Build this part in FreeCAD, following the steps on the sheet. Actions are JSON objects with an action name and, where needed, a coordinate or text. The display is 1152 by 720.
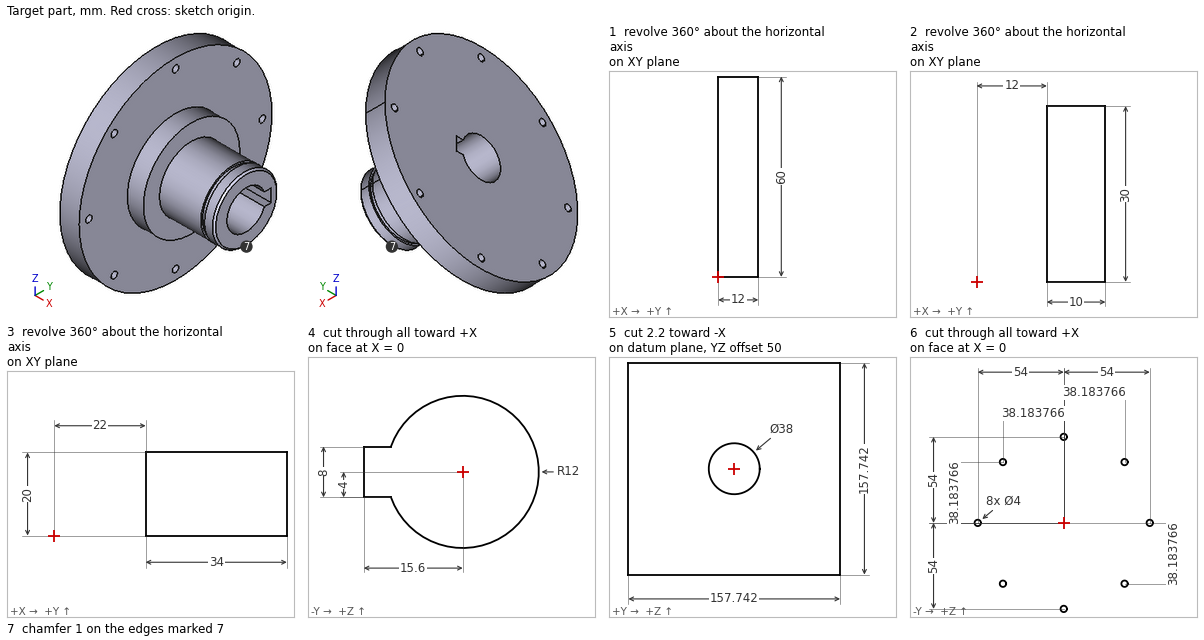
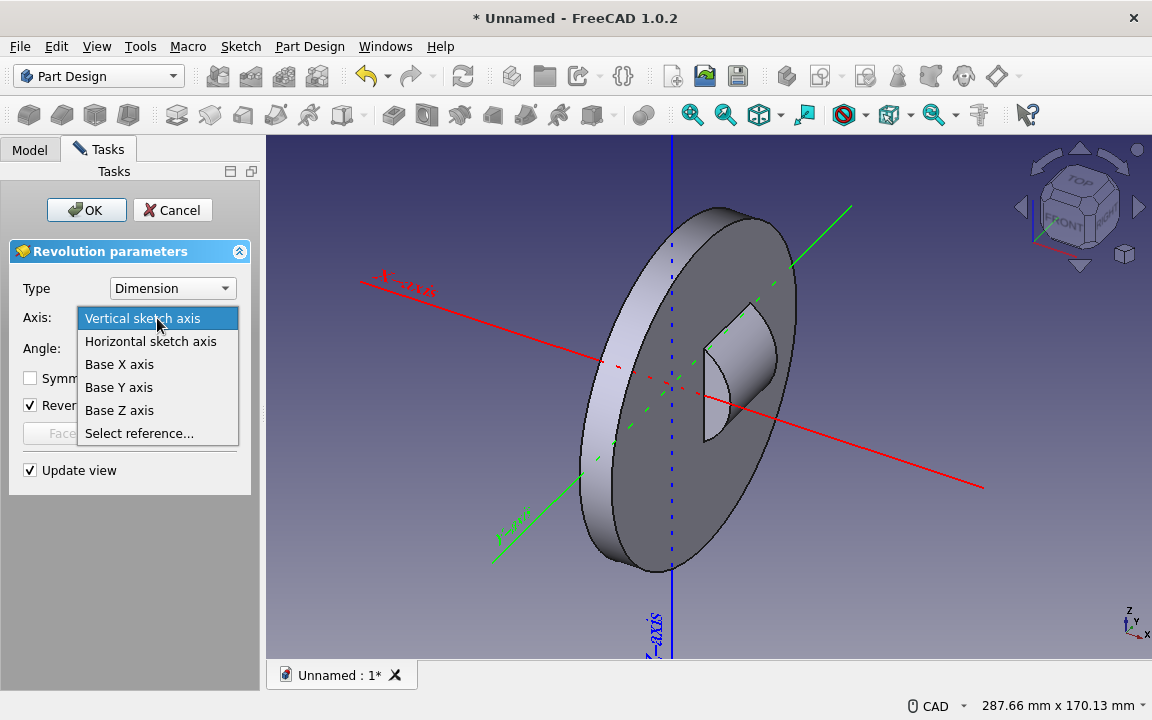
{"action": "left_click", "coordinate": [156, 342]}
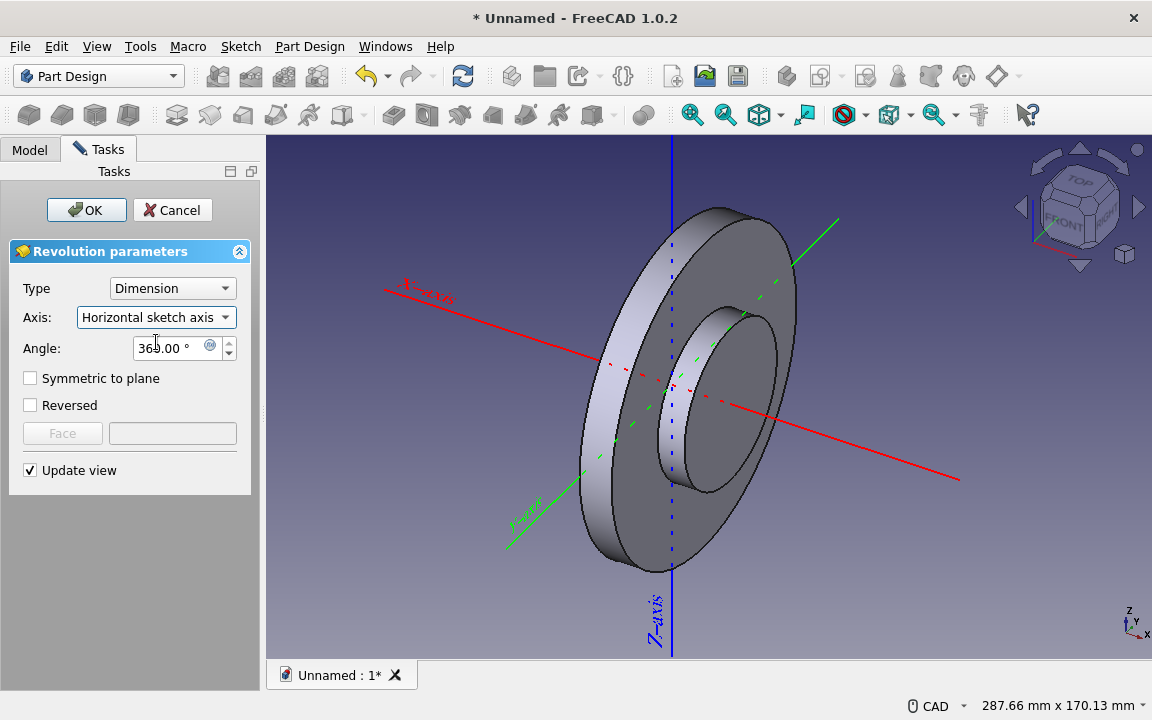
{"action": "left_click", "coordinate": [87, 210]}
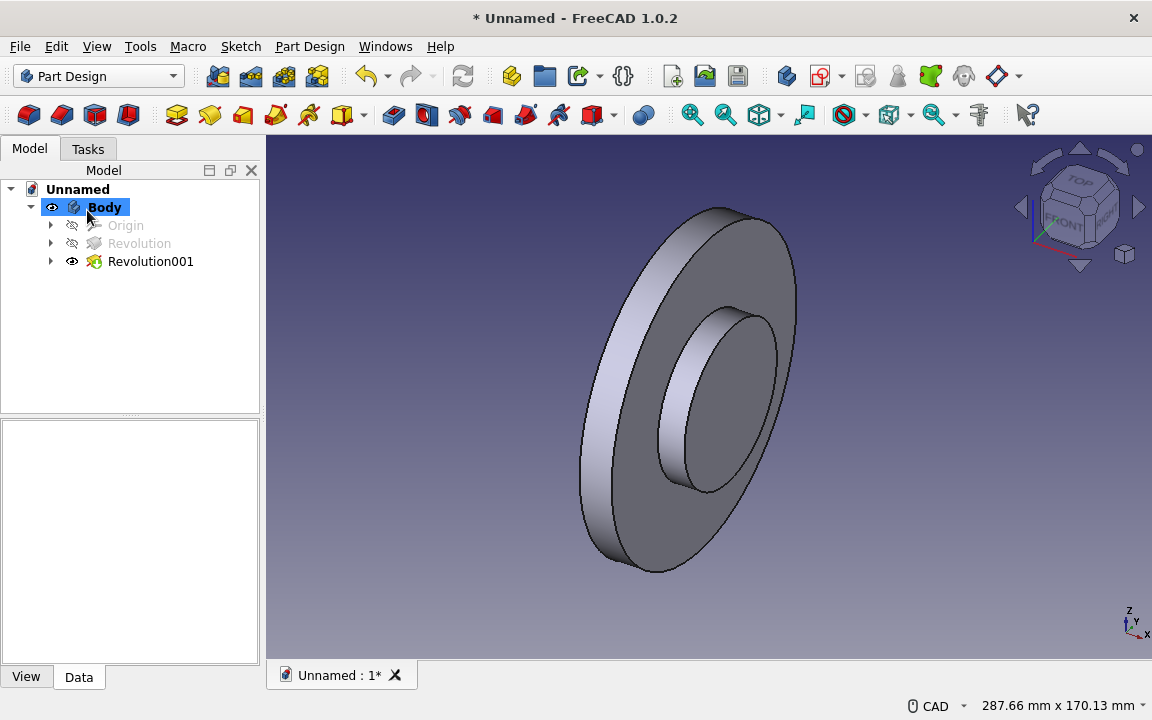
{"action": "left_click", "coordinate": [820, 76]}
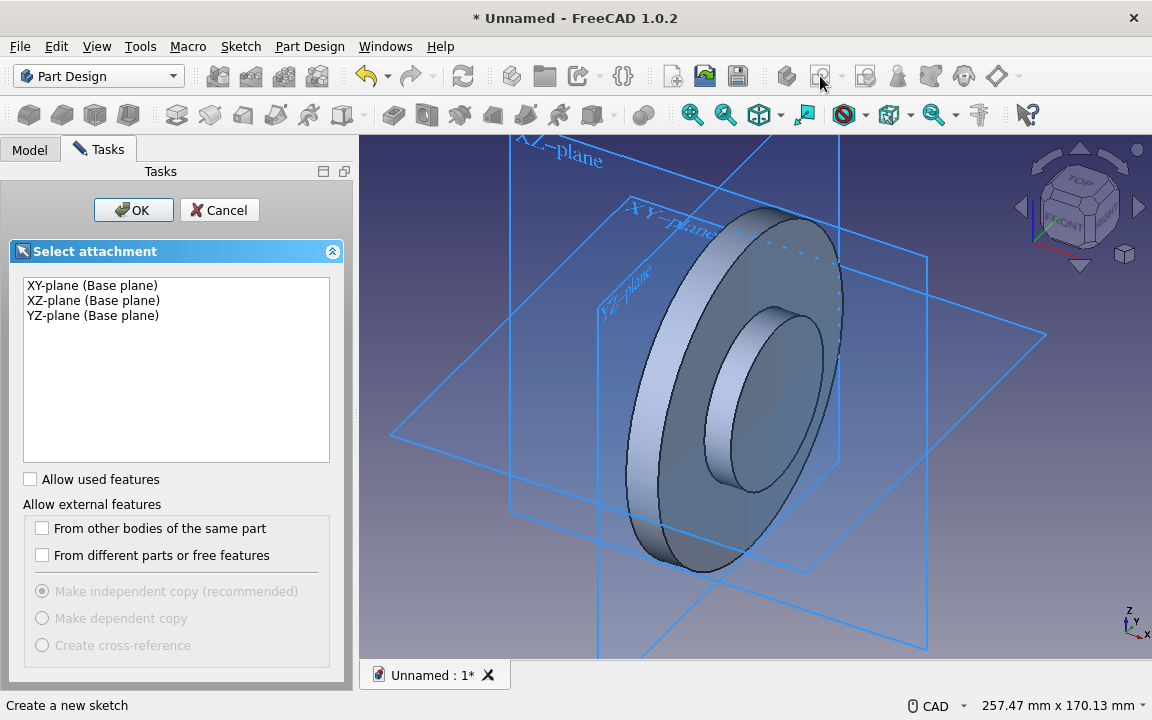
{"action": "left_click", "coordinate": [84, 286]}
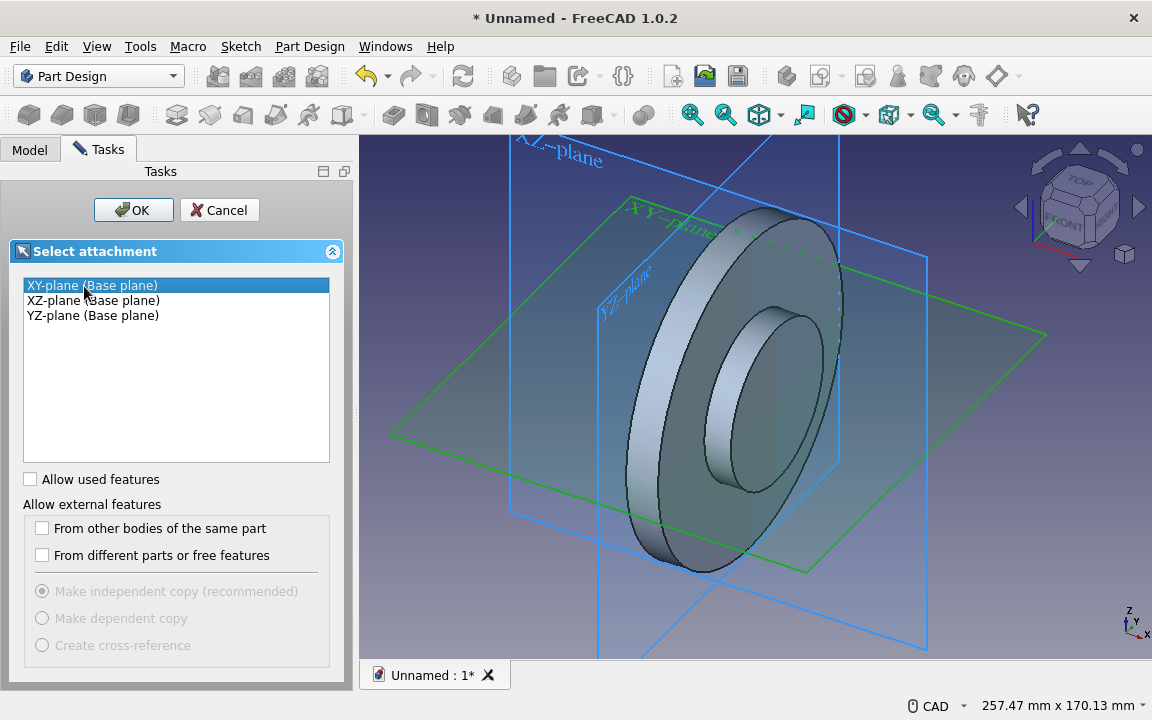
{"action": "left_click", "coordinate": [134, 210]}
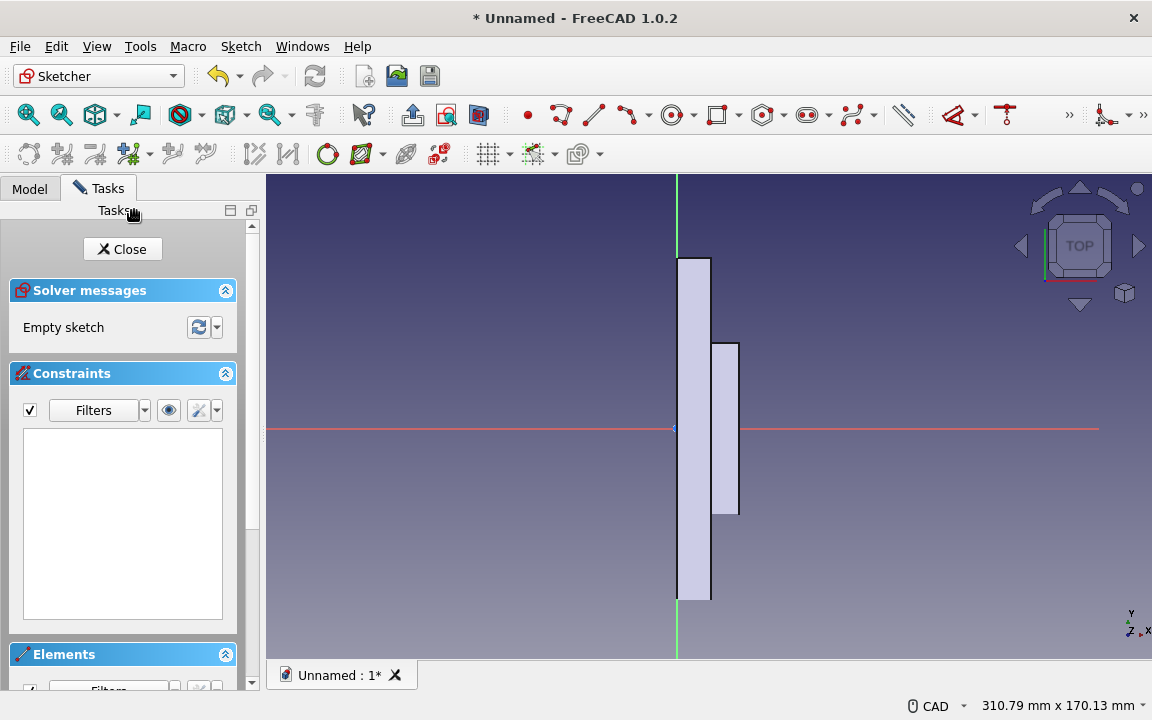
{"action": "left_click", "coordinate": [479, 116]}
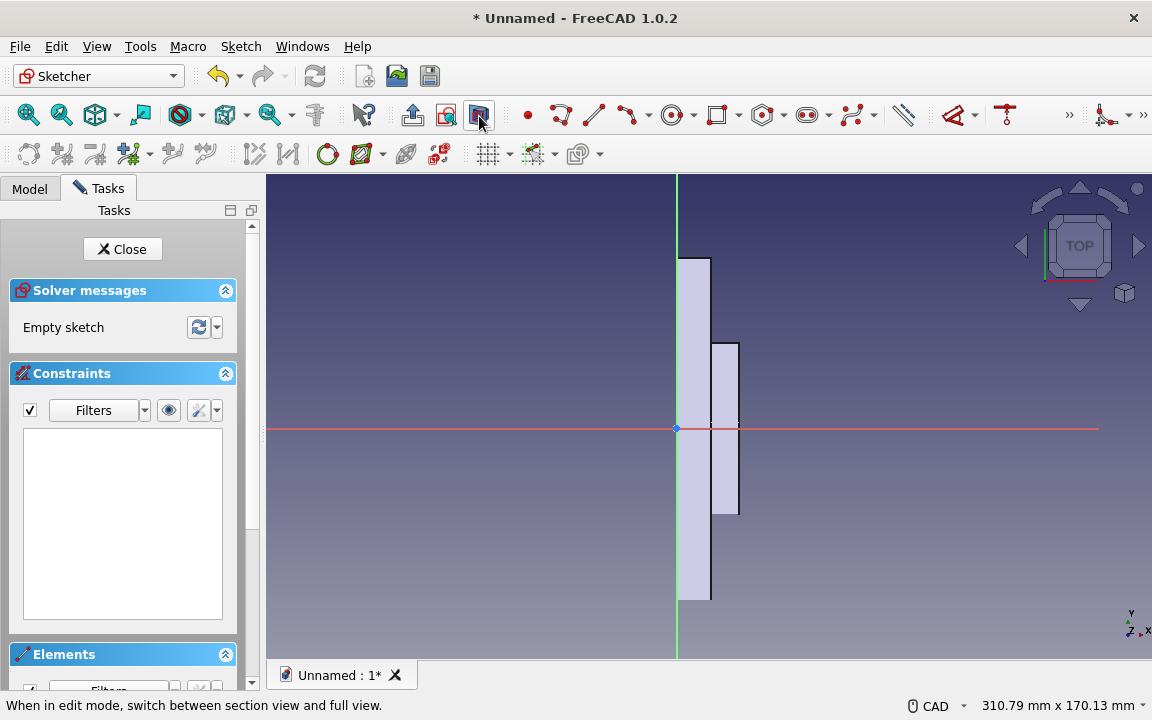
{"action": "scroll", "coordinate": [806, 393], "scroll_direction": "up", "scroll_amount": 6}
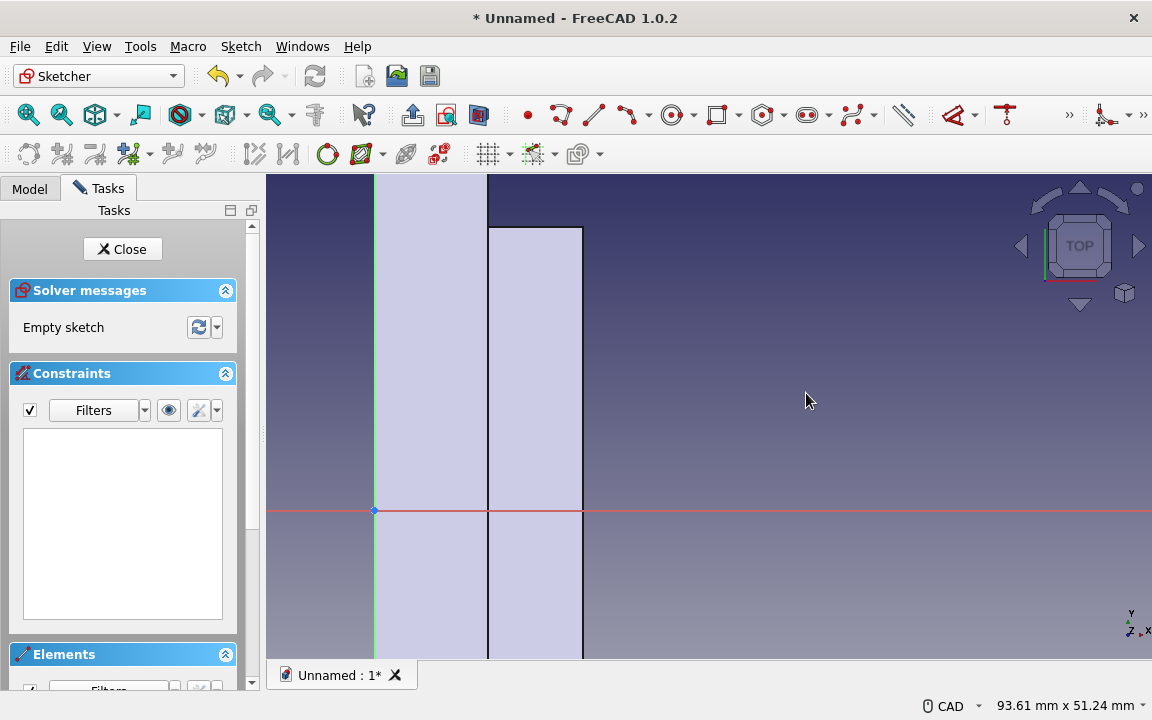
{"action": "left_click", "coordinate": [716, 116]}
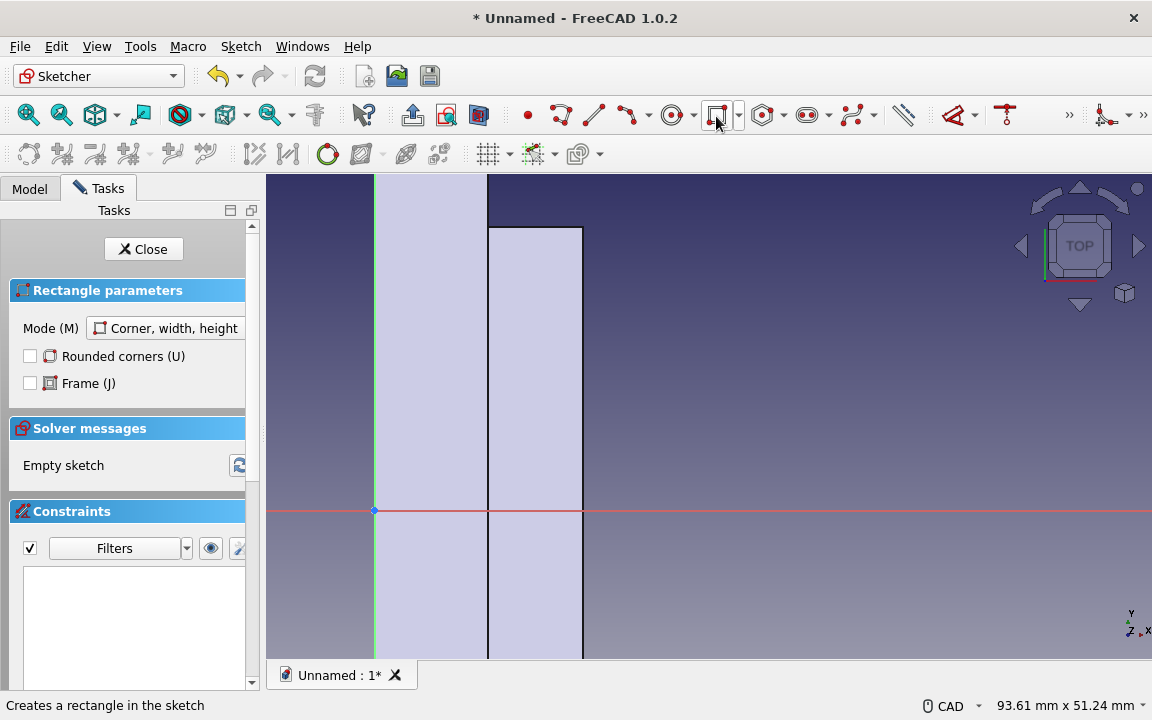
{"action": "left_click", "coordinate": [583, 321]}
{"action": "left_click", "coordinate": [905, 511]}
{"action": "key", "text": "Escape"}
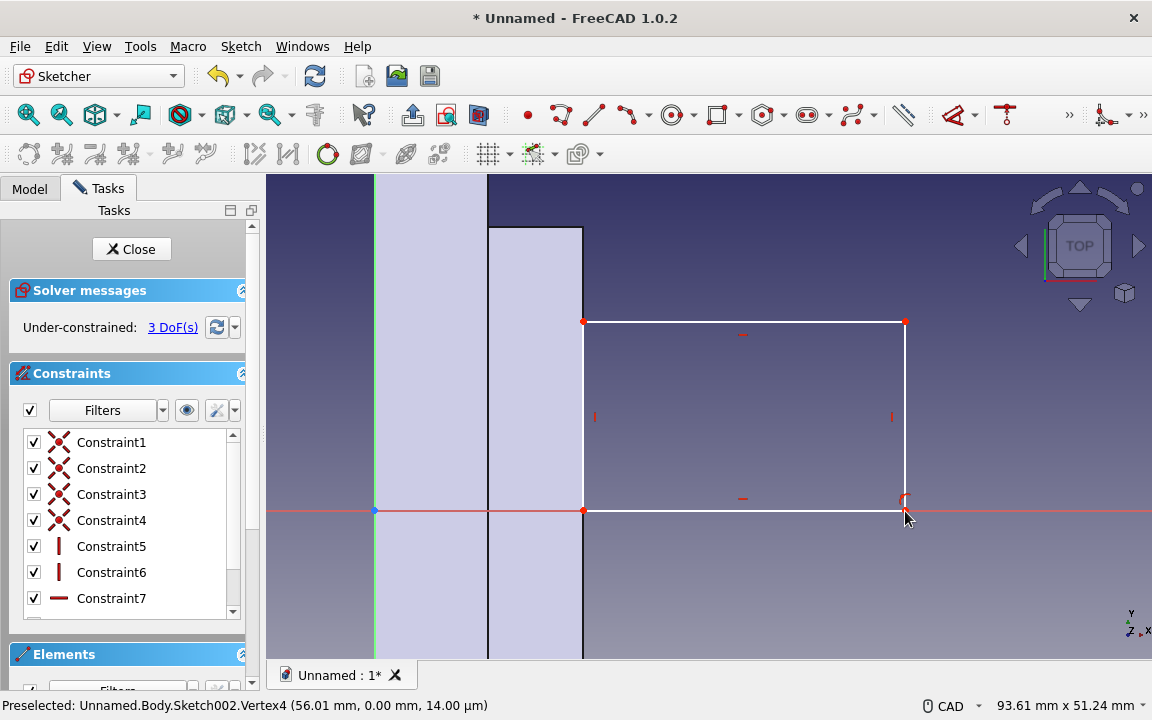
{"action": "left_click", "coordinate": [952, 116]}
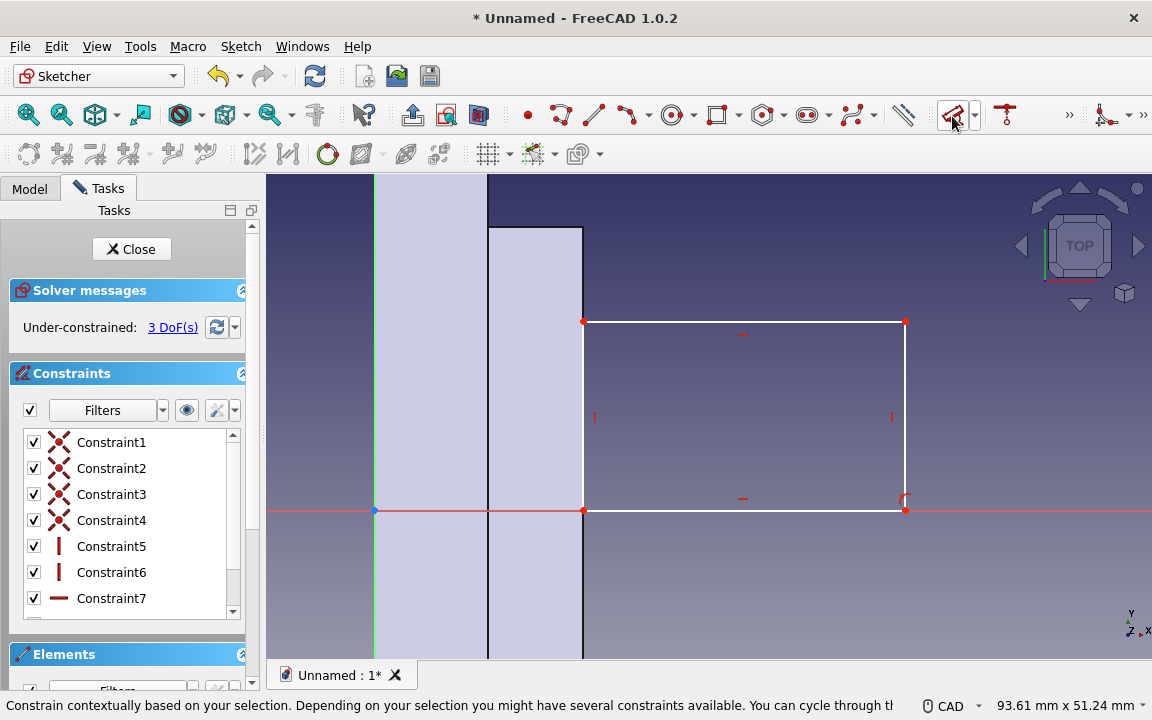
{"action": "left_click", "coordinate": [583, 379]}
{"action": "left_click", "coordinate": [549, 416]}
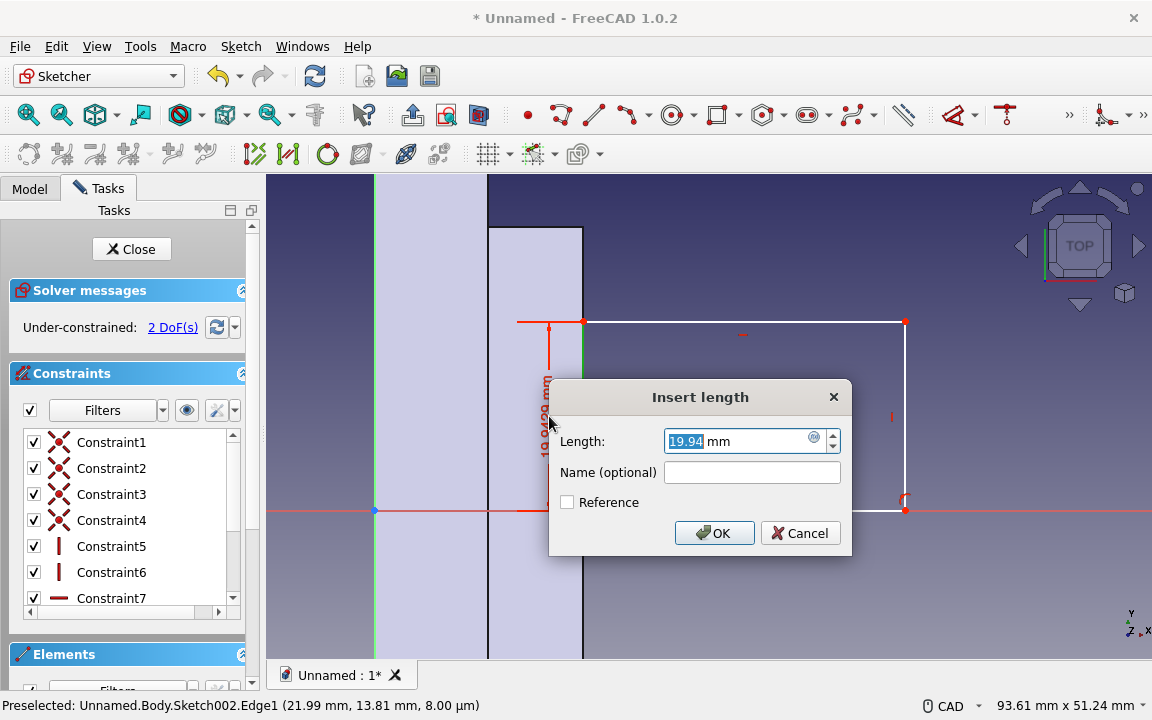
{"action": "type", "text": "20"}
{"action": "key", "text": "Return"}